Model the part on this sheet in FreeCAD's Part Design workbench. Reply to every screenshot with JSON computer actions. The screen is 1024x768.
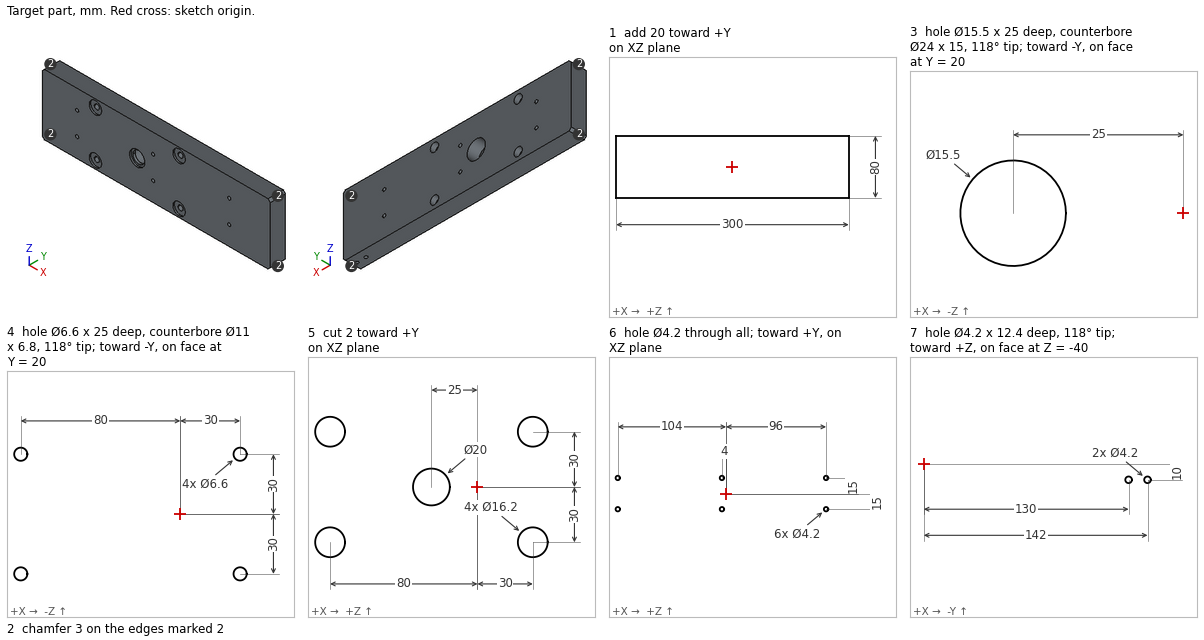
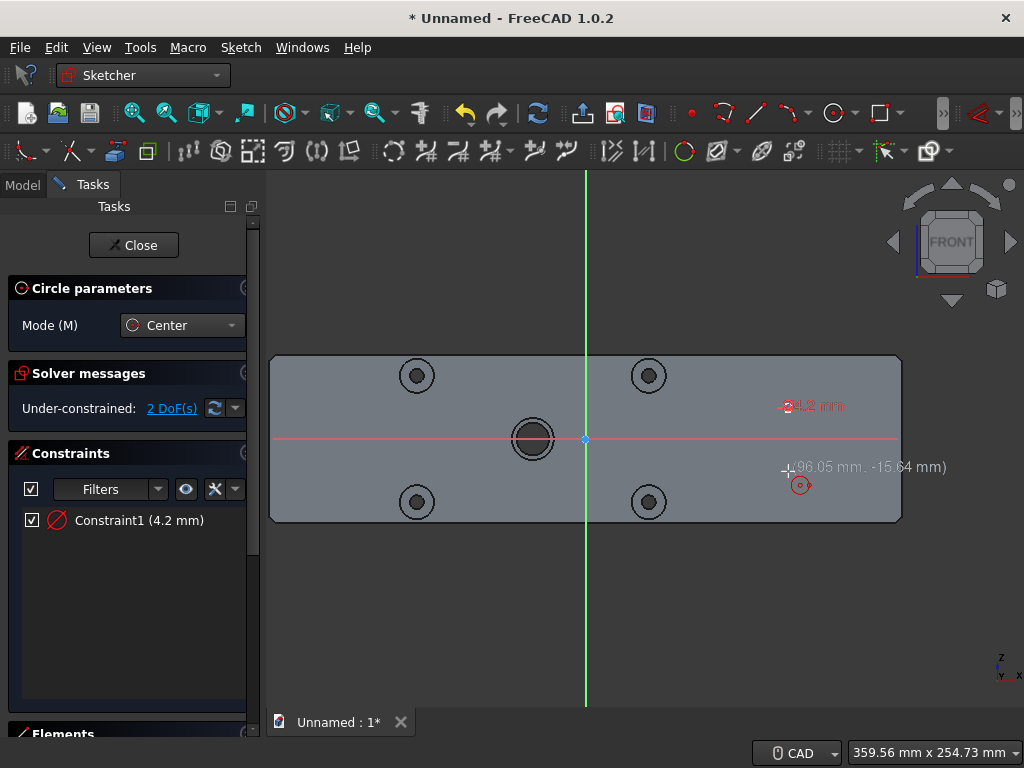
{"action": "left_click", "coordinate": [788, 471]}
{"action": "mouse_move", "coordinate": [791, 468]}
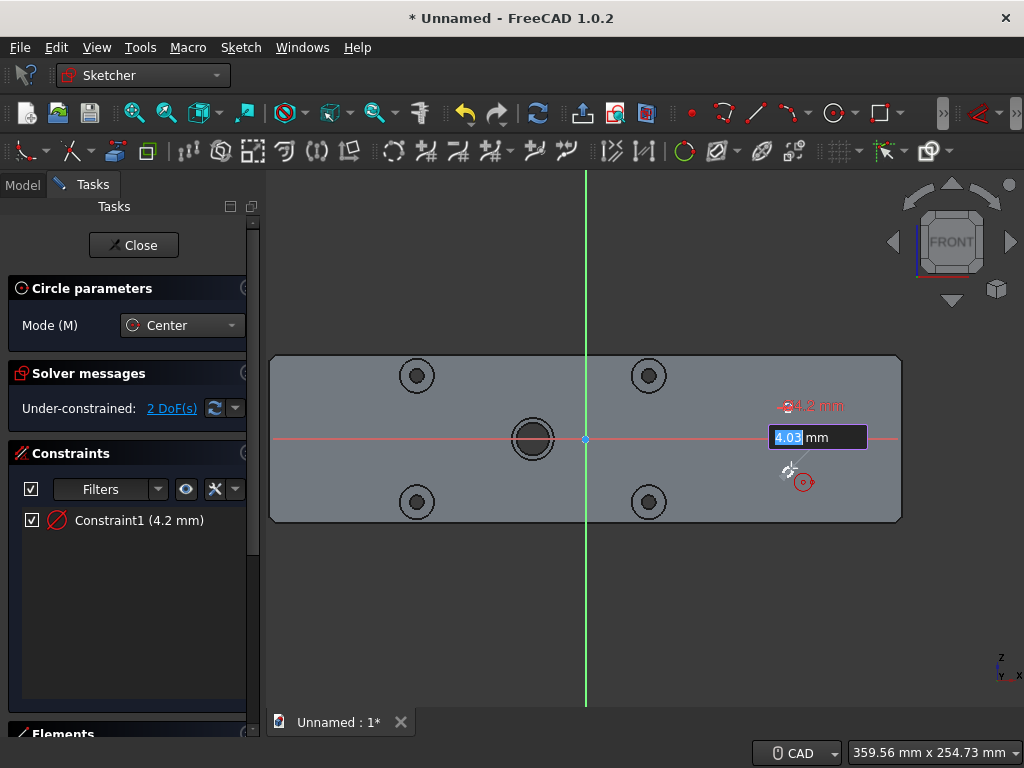
{"action": "type", "text": "4.2"}
{"action": "key", "text": "Return"}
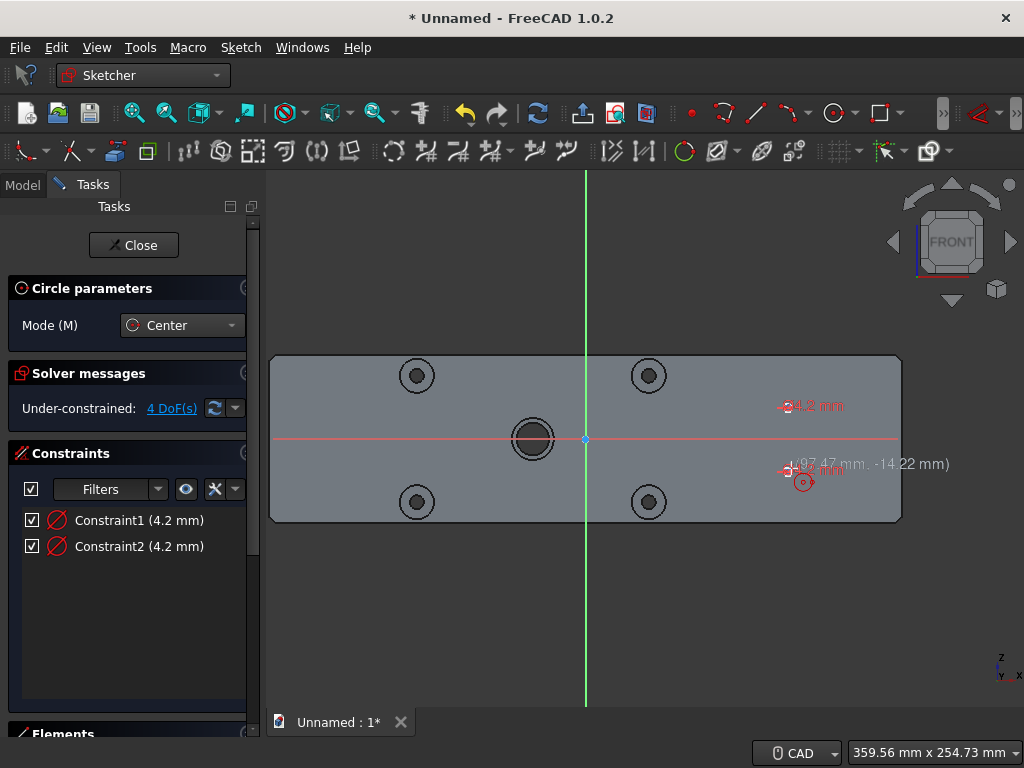
{"action": "scroll", "coordinate": [577, 407], "scroll_direction": "up", "scroll_amount": 9}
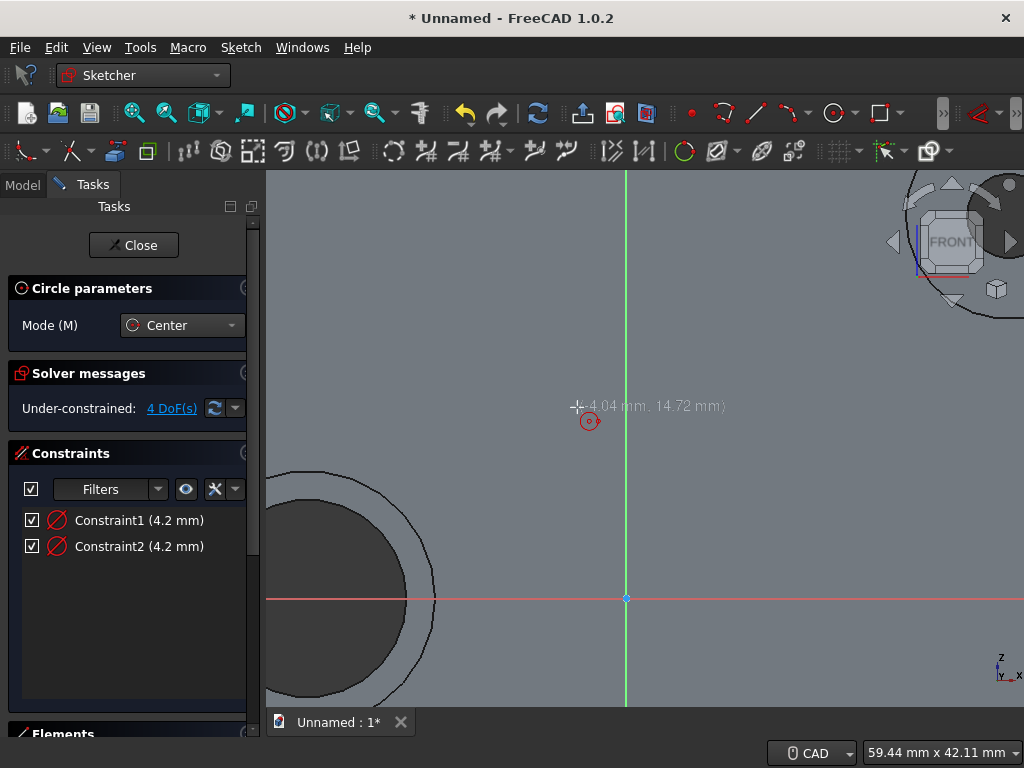
{"action": "scroll", "coordinate": [577, 407], "scroll_direction": "down", "scroll_amount": 9}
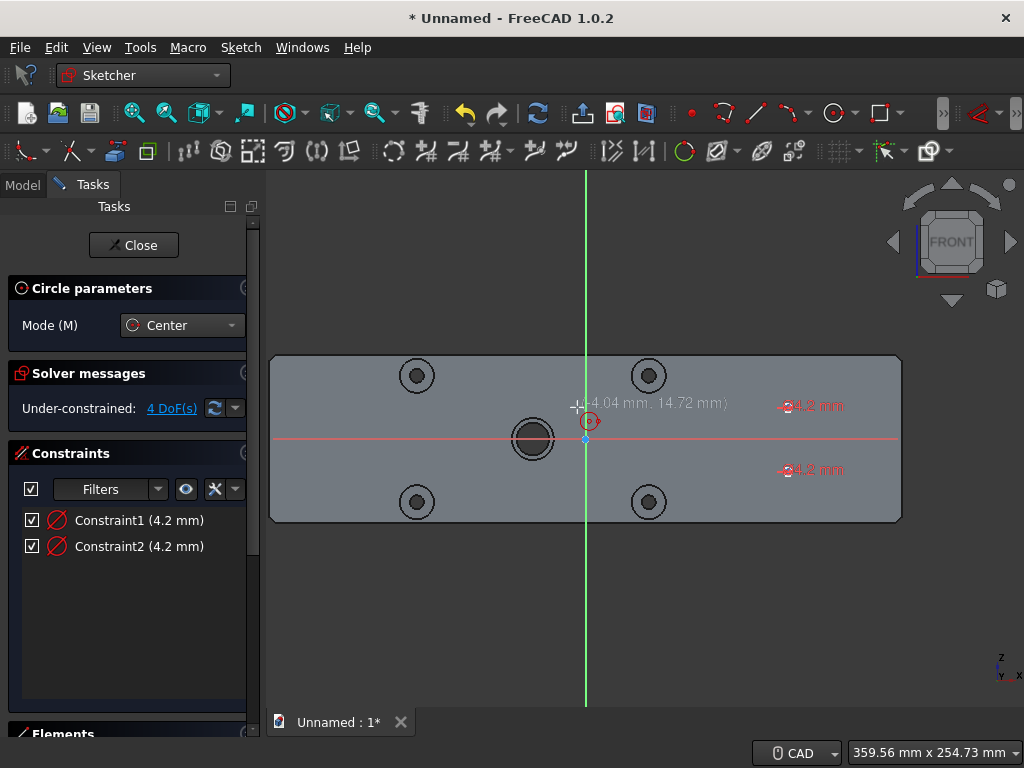
{"action": "scroll", "coordinate": [577, 407], "scroll_direction": "up", "scroll_amount": 4}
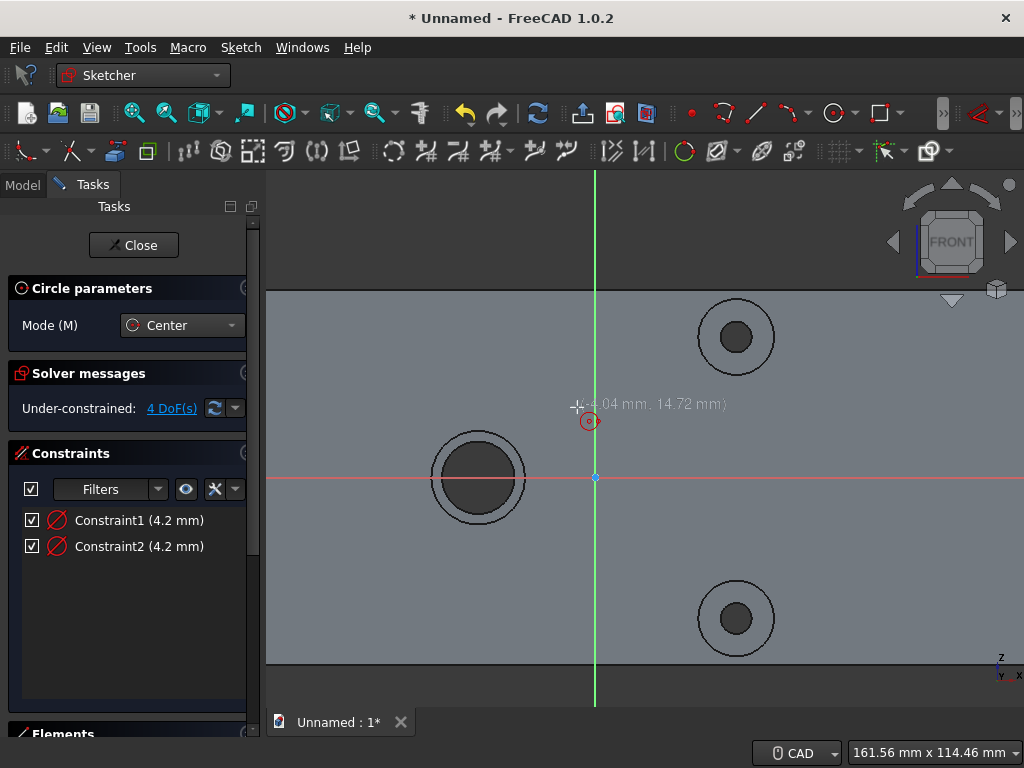
{"action": "left_click", "coordinate": [577, 407]}
{"action": "mouse_move", "coordinate": [570, 400]}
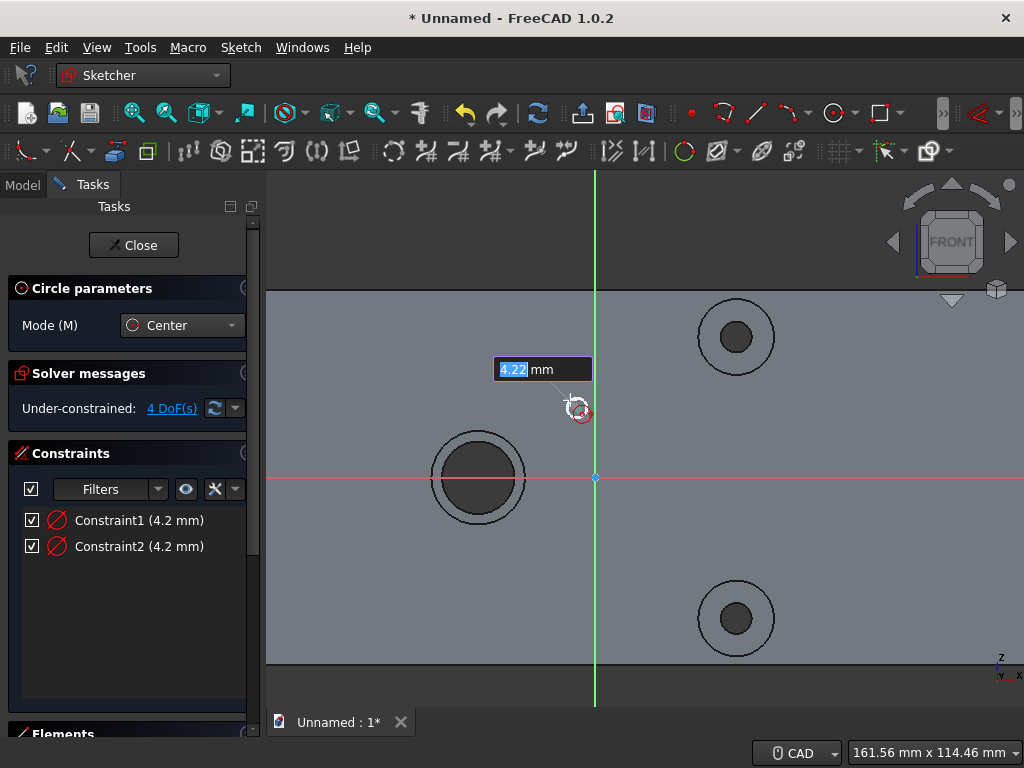
{"action": "type", "text": "4.2"}
{"action": "key", "text": "Return"}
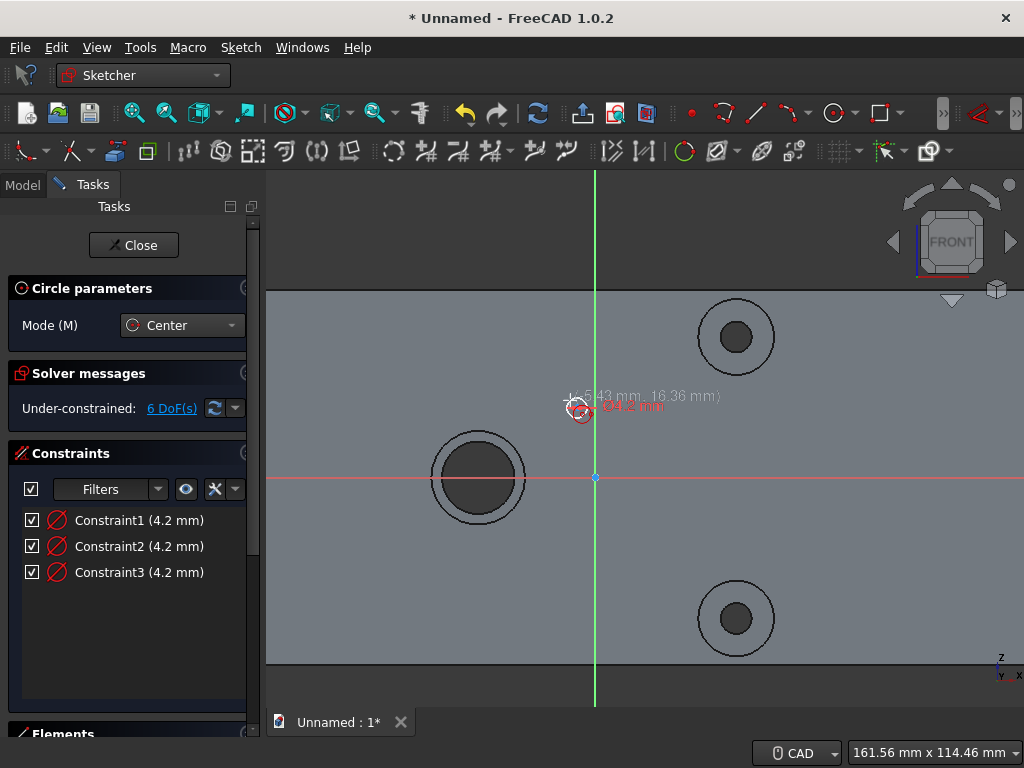
{"action": "scroll", "coordinate": [577, 548], "scroll_direction": "up", "scroll_amount": 5}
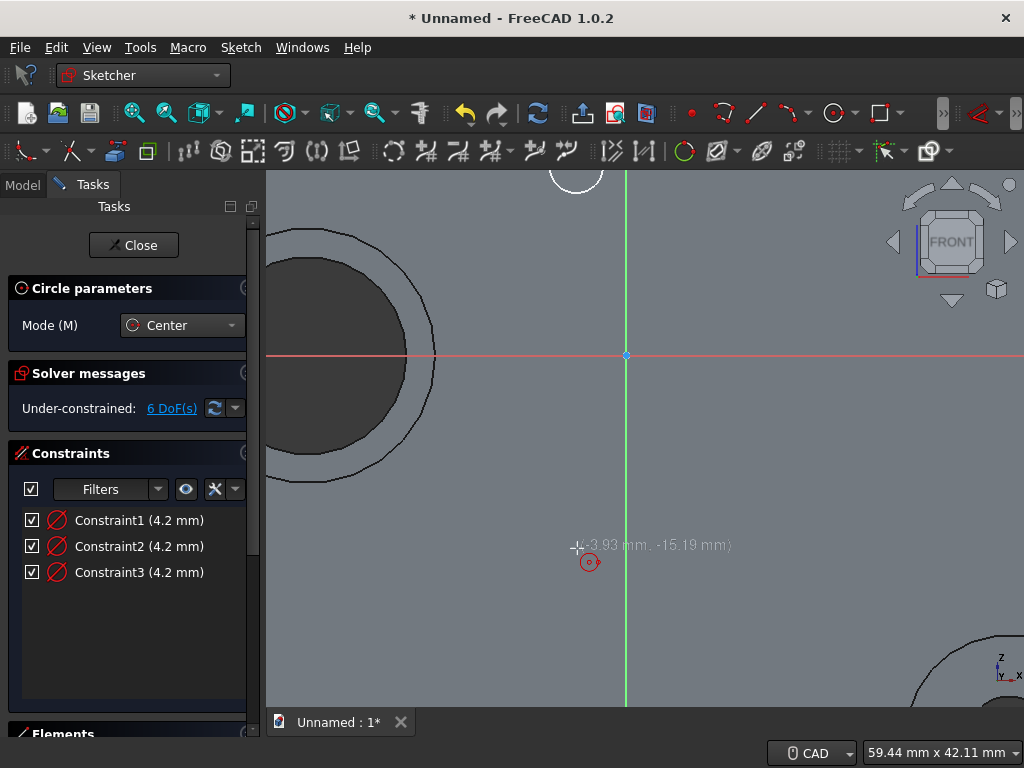
{"action": "scroll", "coordinate": [577, 455], "scroll_direction": "down", "scroll_amount": 9}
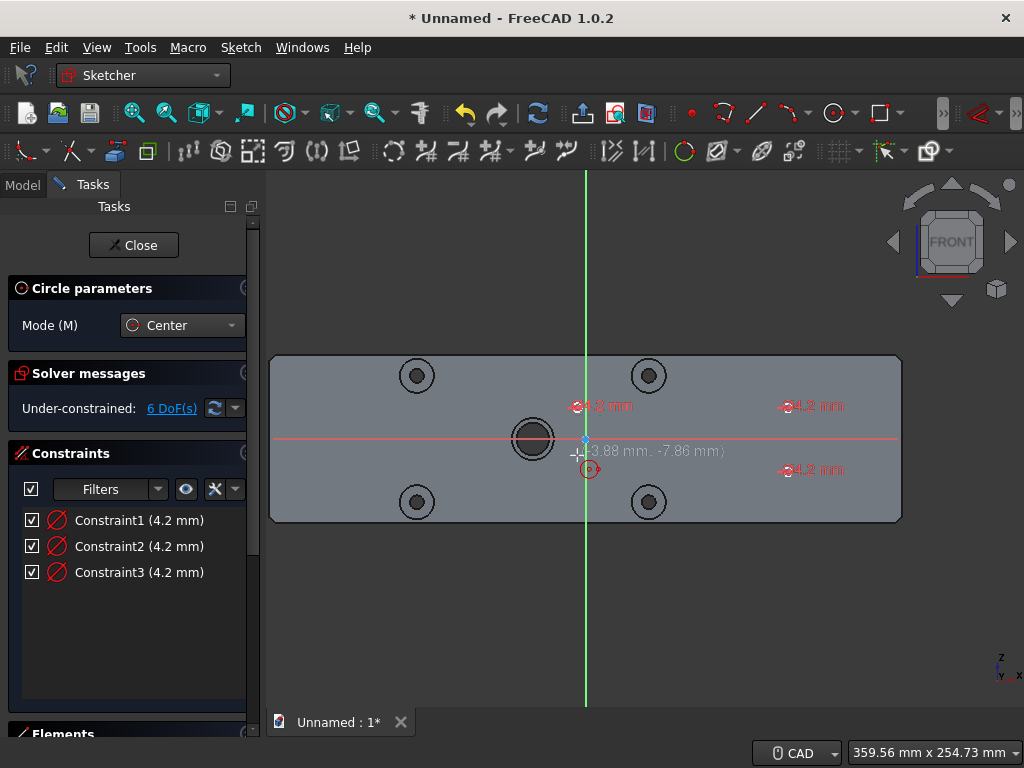
{"action": "scroll", "coordinate": [577, 471], "scroll_direction": "up", "scroll_amount": 4}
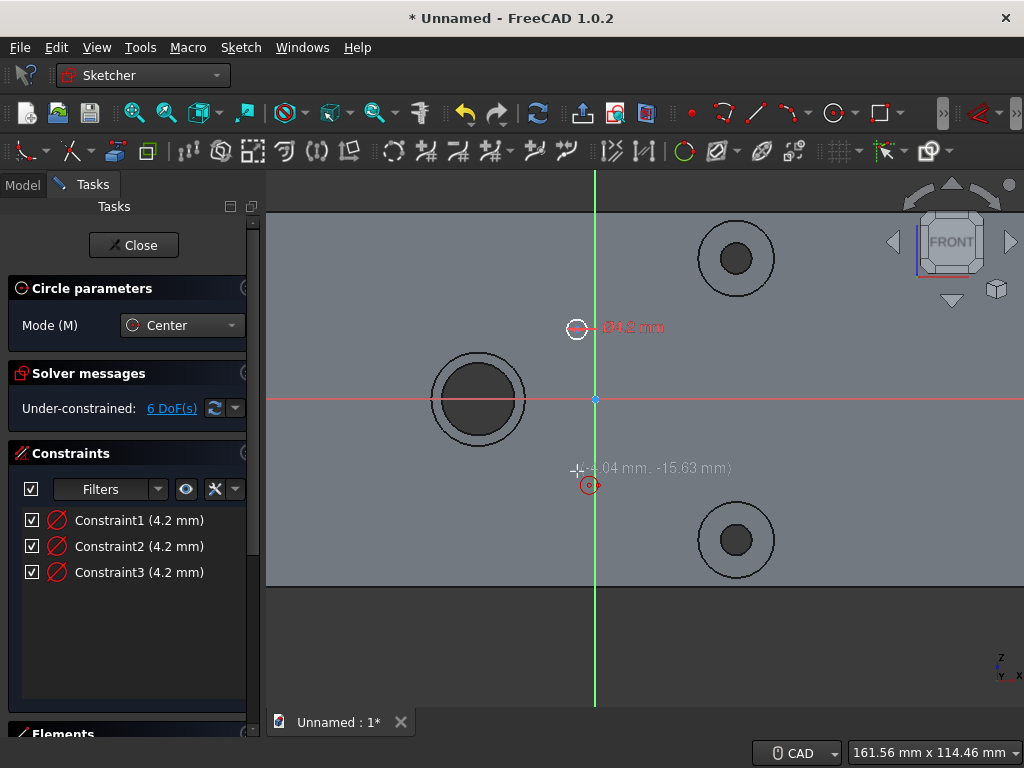
{"action": "left_click", "coordinate": [577, 470]}
{"action": "mouse_move", "coordinate": [570, 463]}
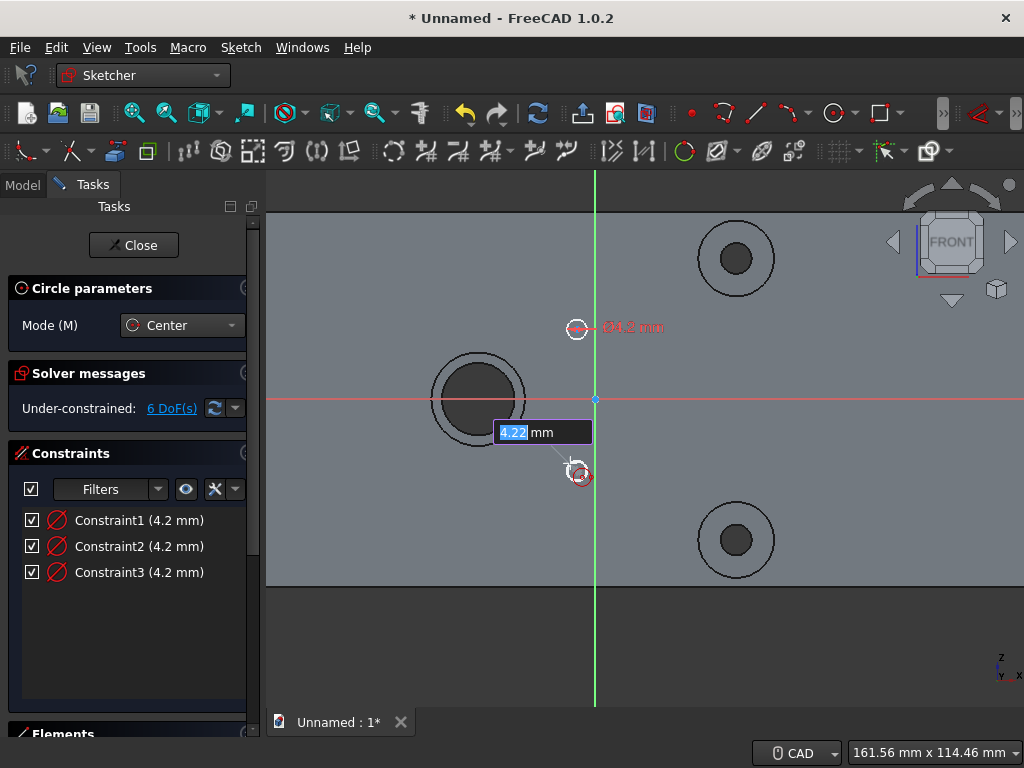
{"action": "type", "text": "4.2"}
{"action": "key", "text": "Return"}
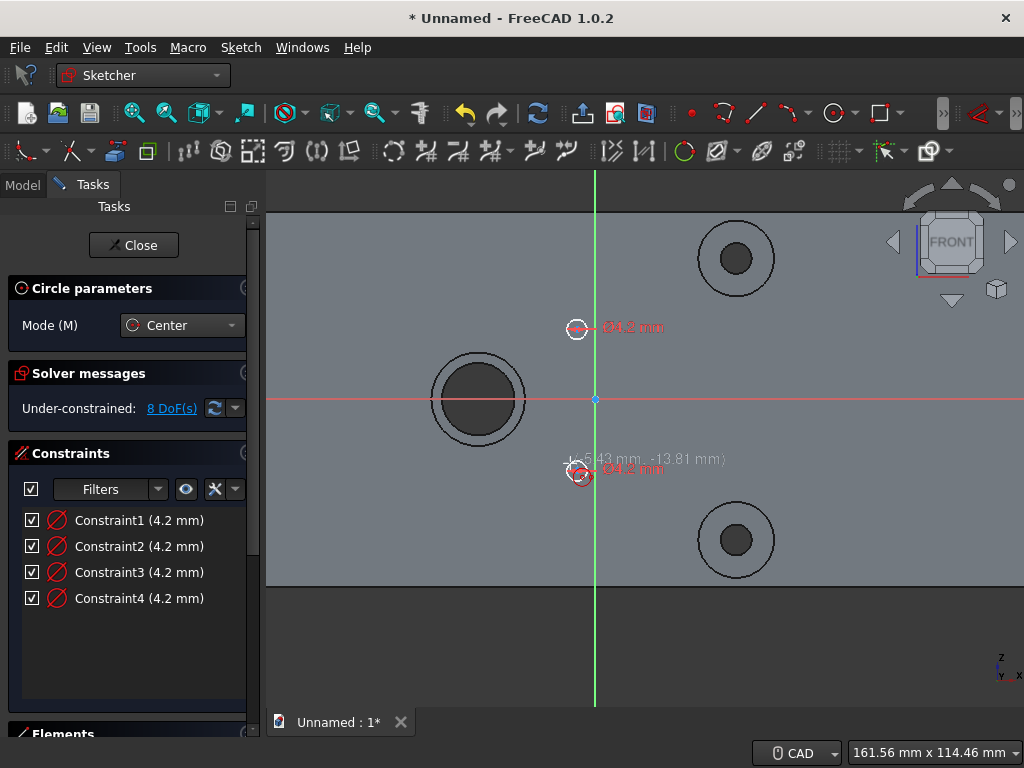
{"action": "scroll", "coordinate": [576, 471], "scroll_direction": "down", "scroll_amount": 4}